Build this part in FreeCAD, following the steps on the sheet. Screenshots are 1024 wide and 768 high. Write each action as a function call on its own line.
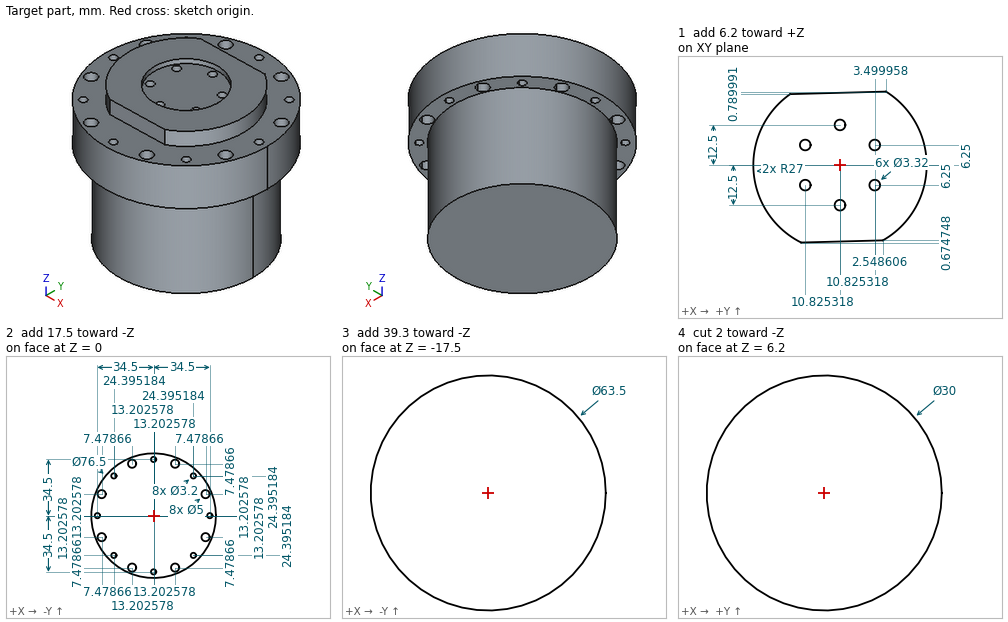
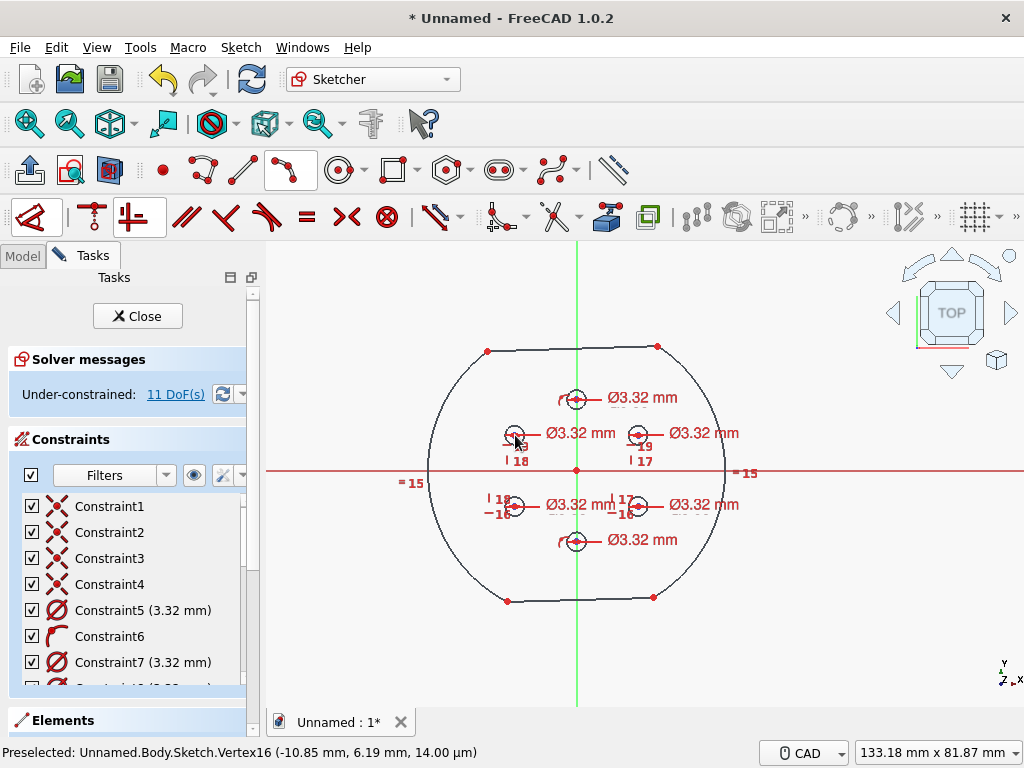
key(d)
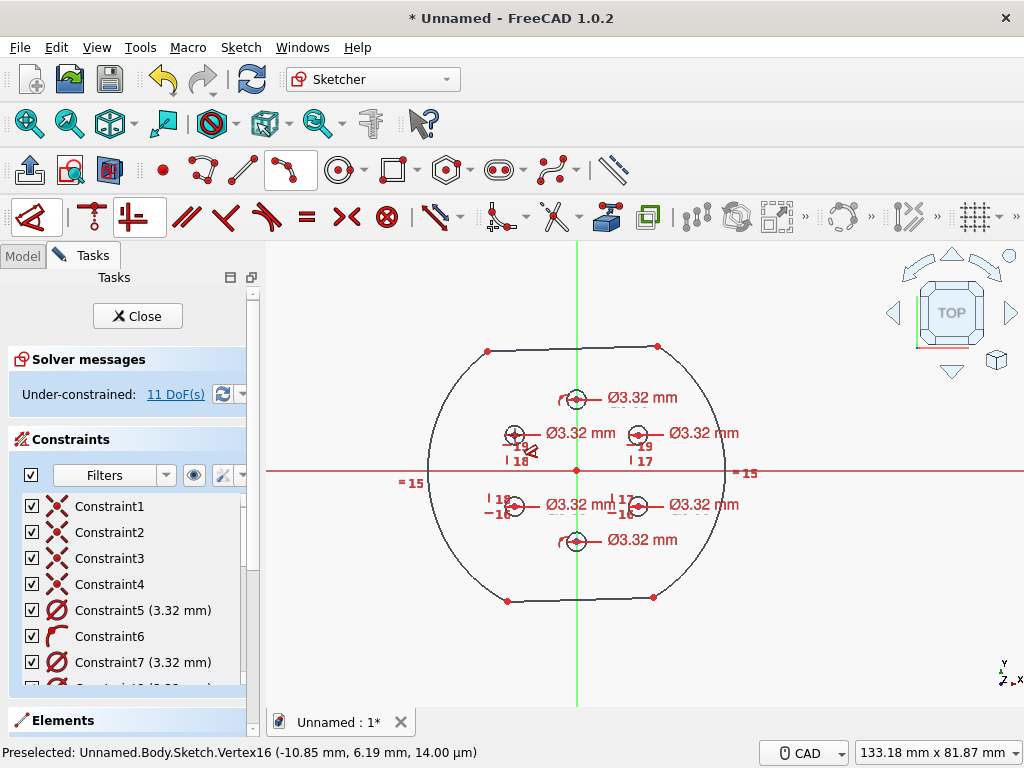
click(436, 423)
click(406, 413)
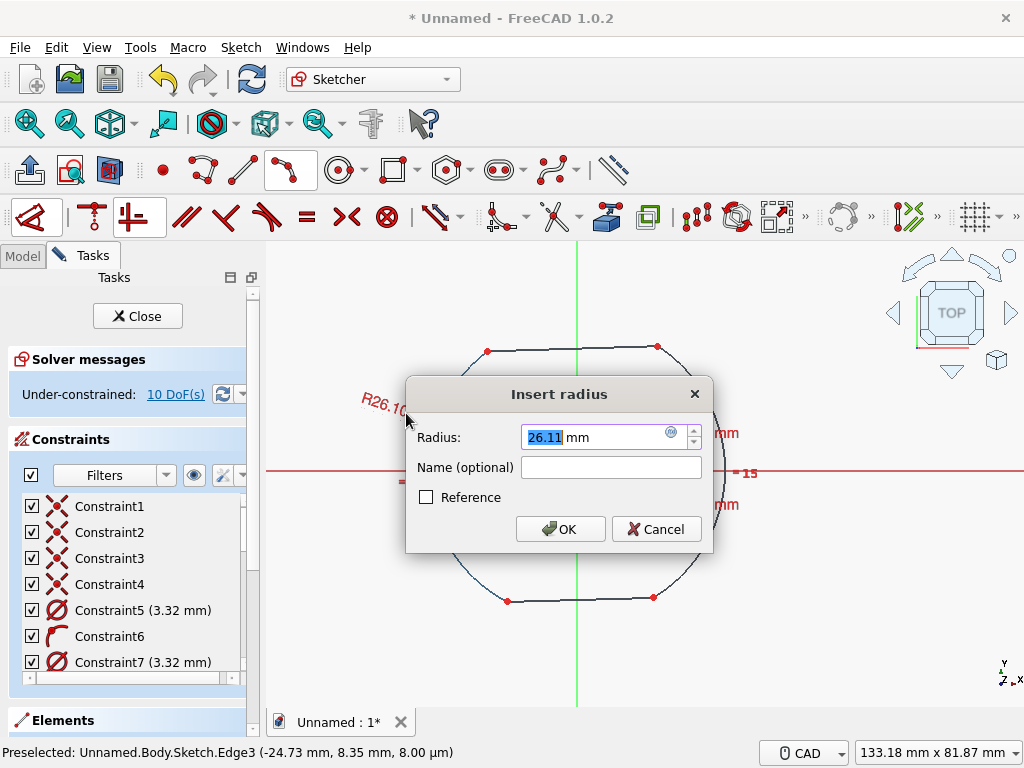
text(27)
key(Return)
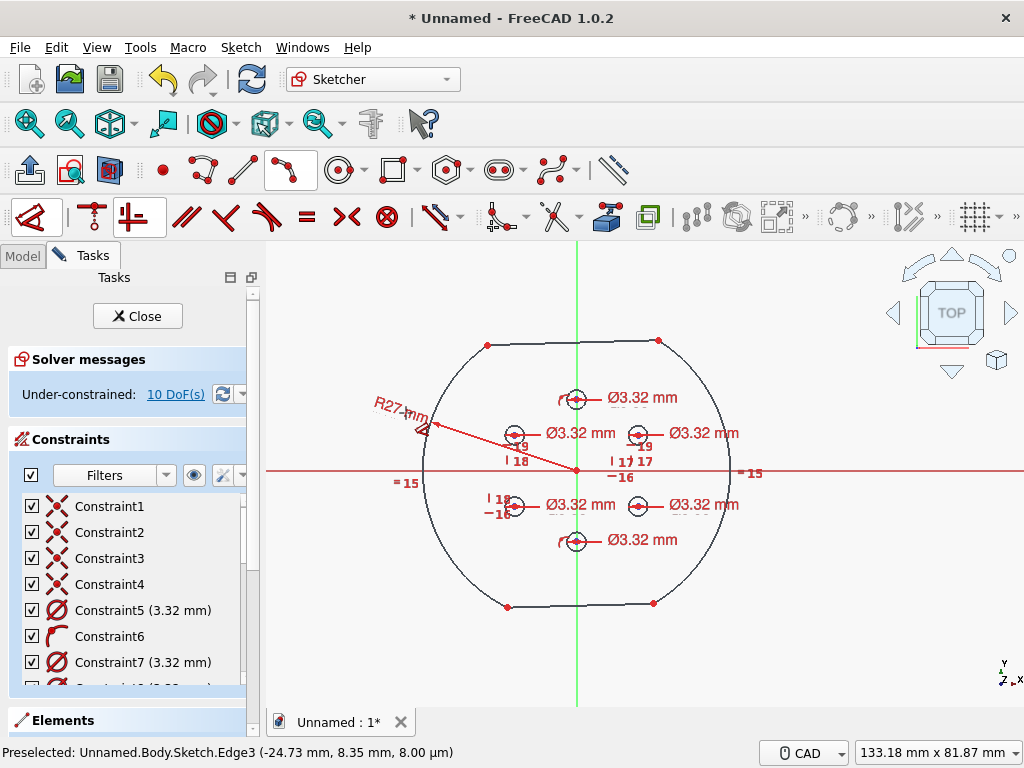
click(577, 542)
click(543, 506)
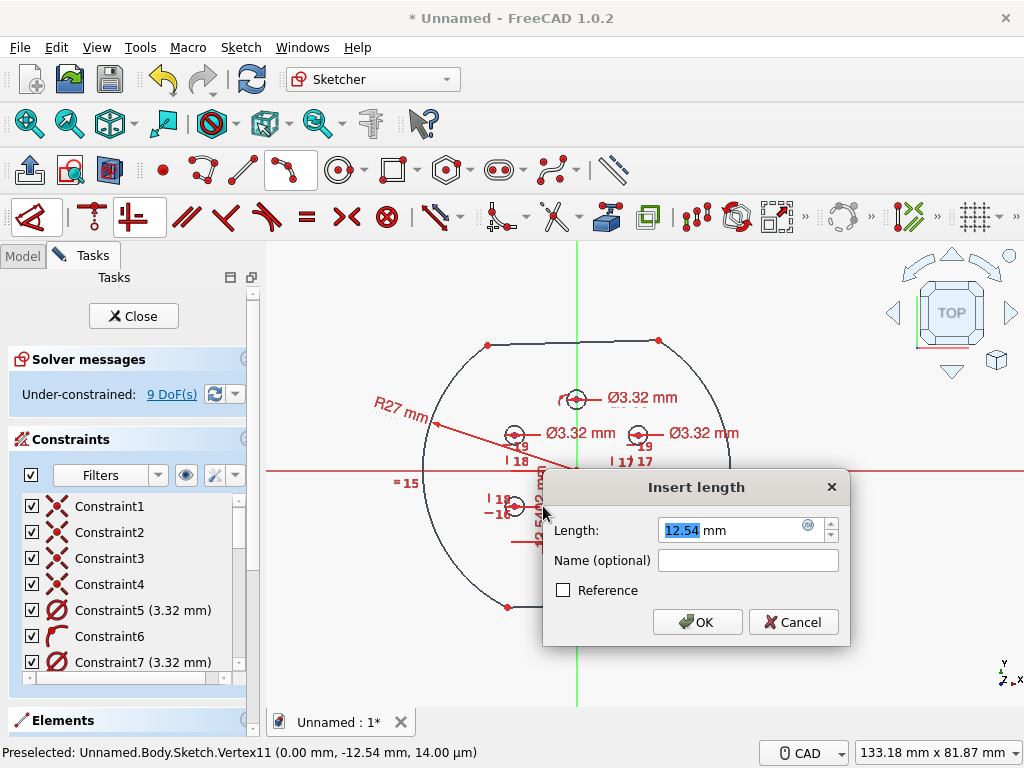
text(12.5)
key(Return)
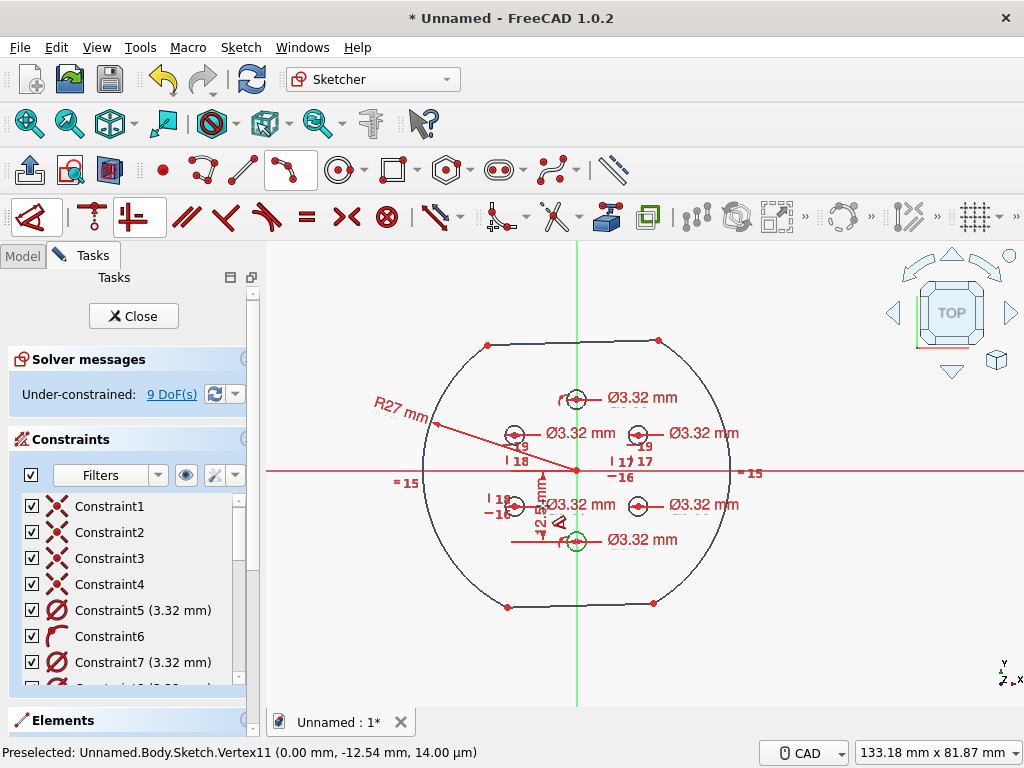
click(638, 507)
click(672, 489)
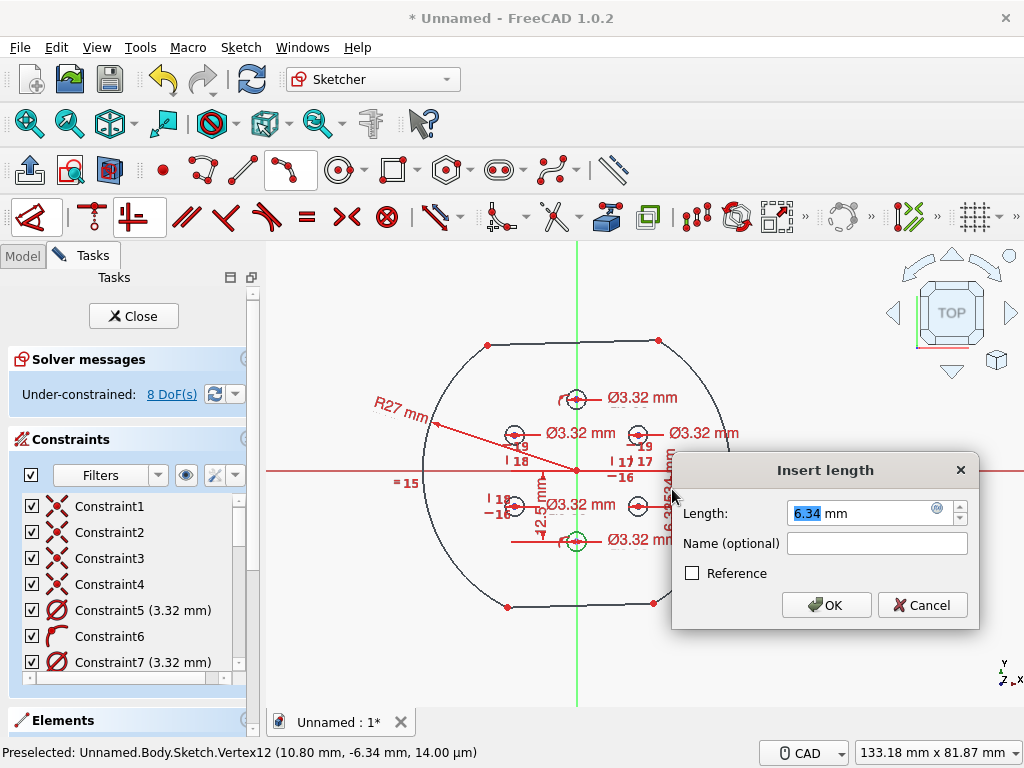
text(6.25)
key(Return)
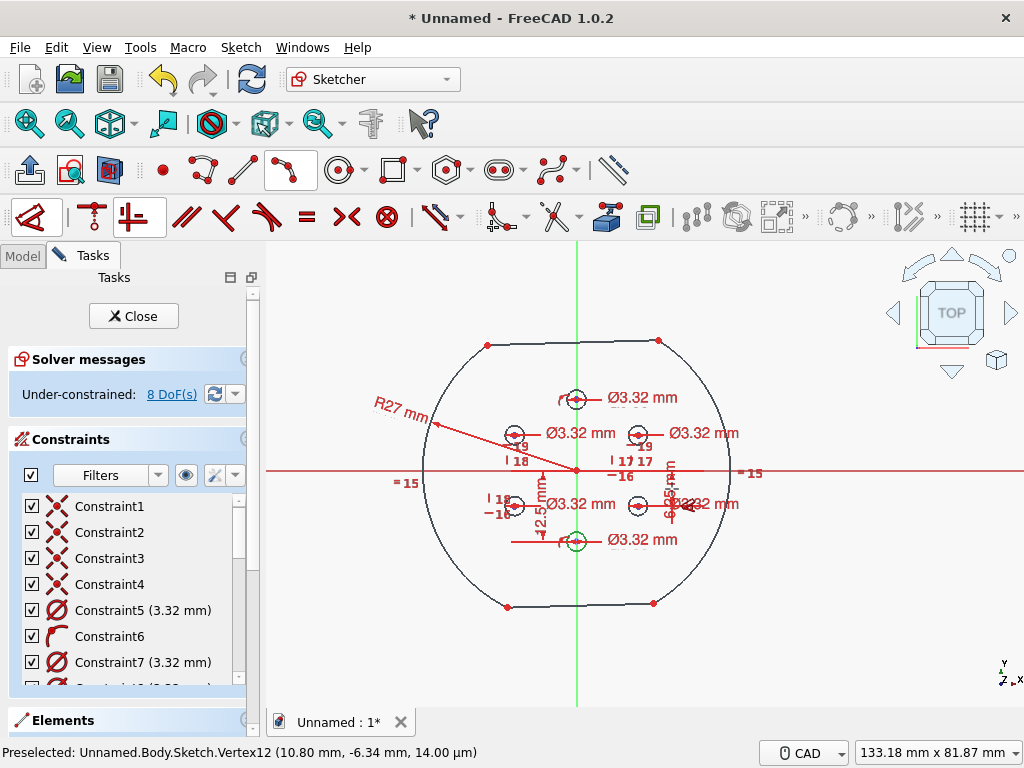
click(638, 435)
click(672, 453)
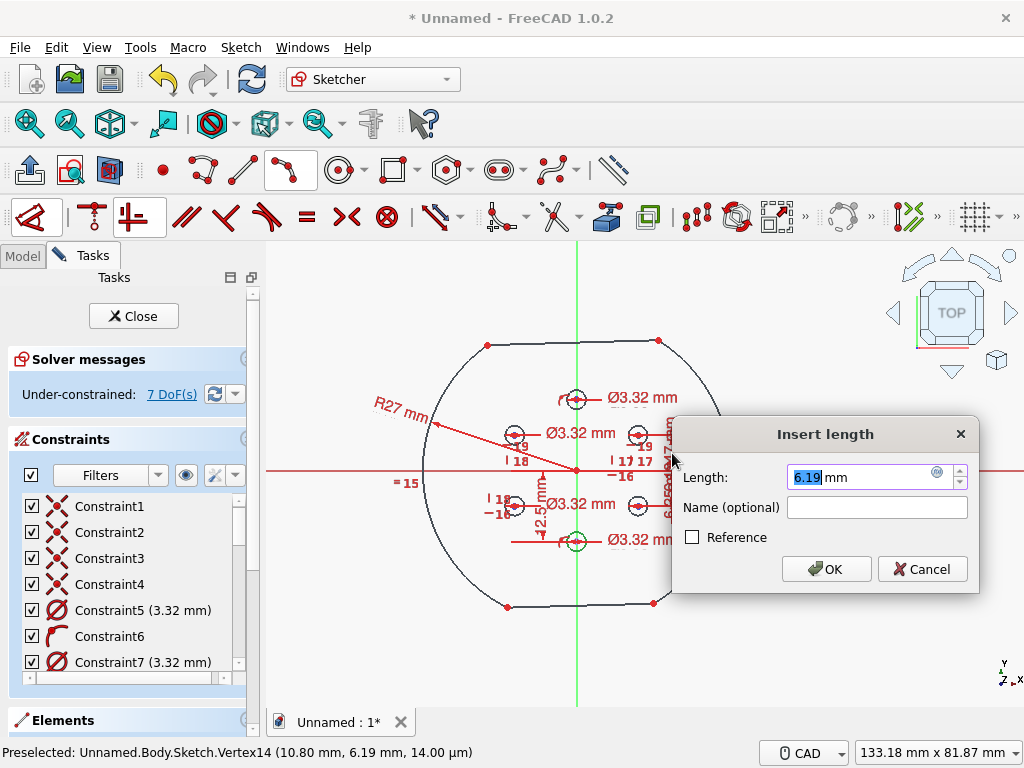
text(6.25)
key(Return)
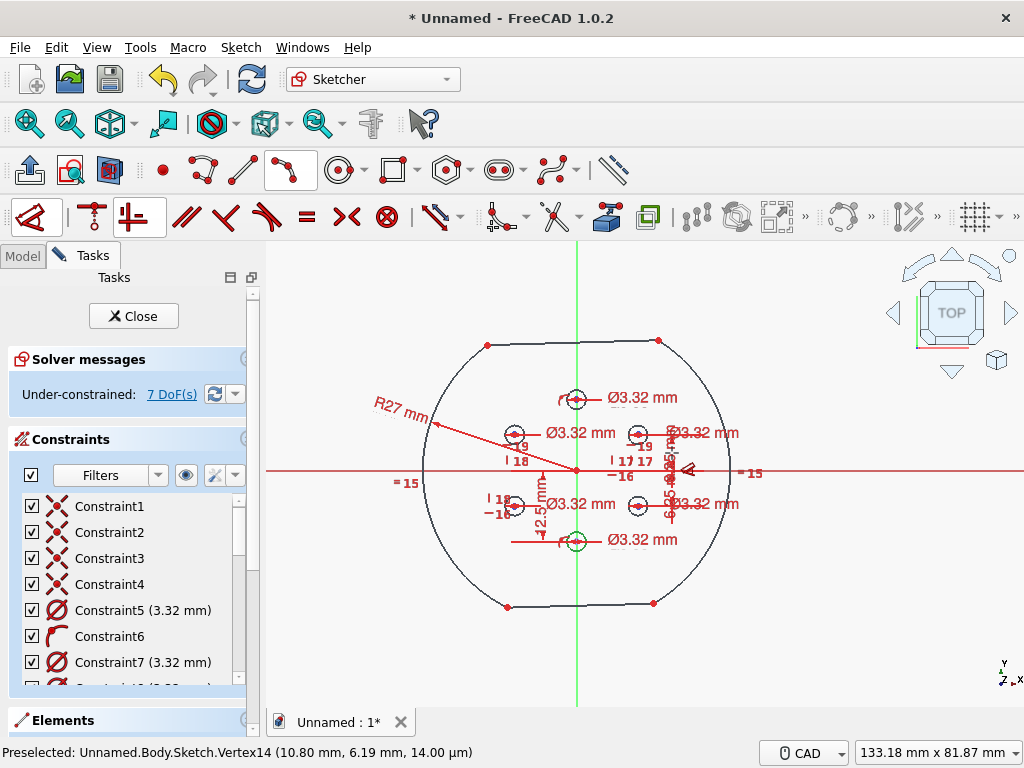
click(577, 400)
click(543, 435)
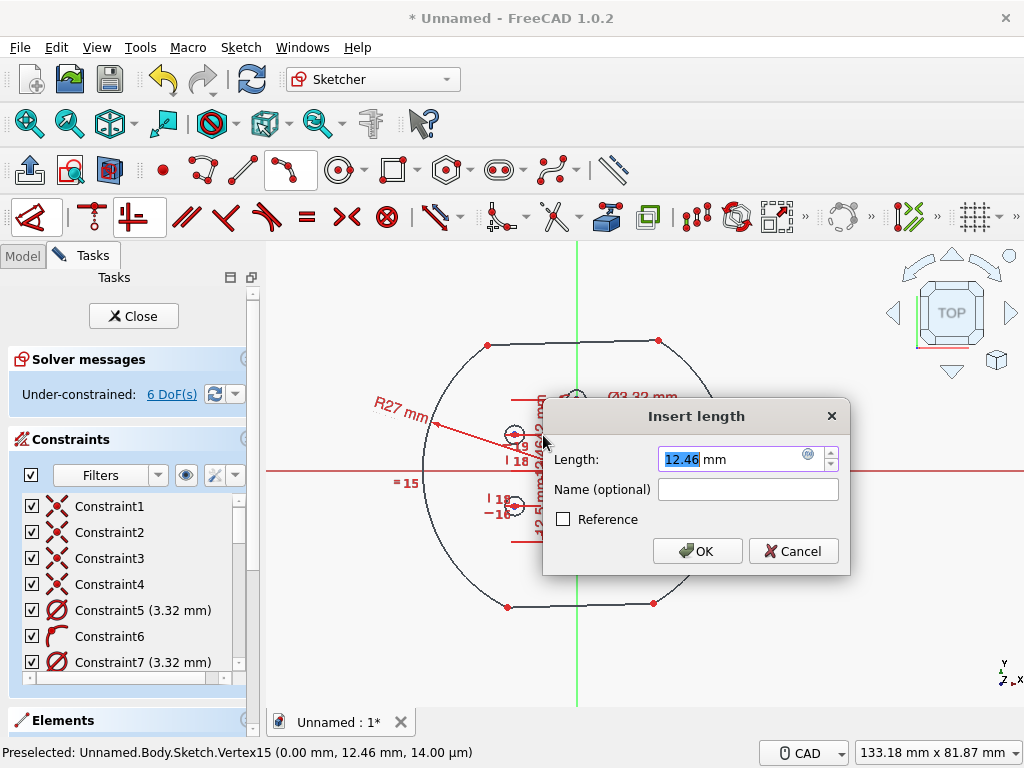
text(12.5)
key(Return)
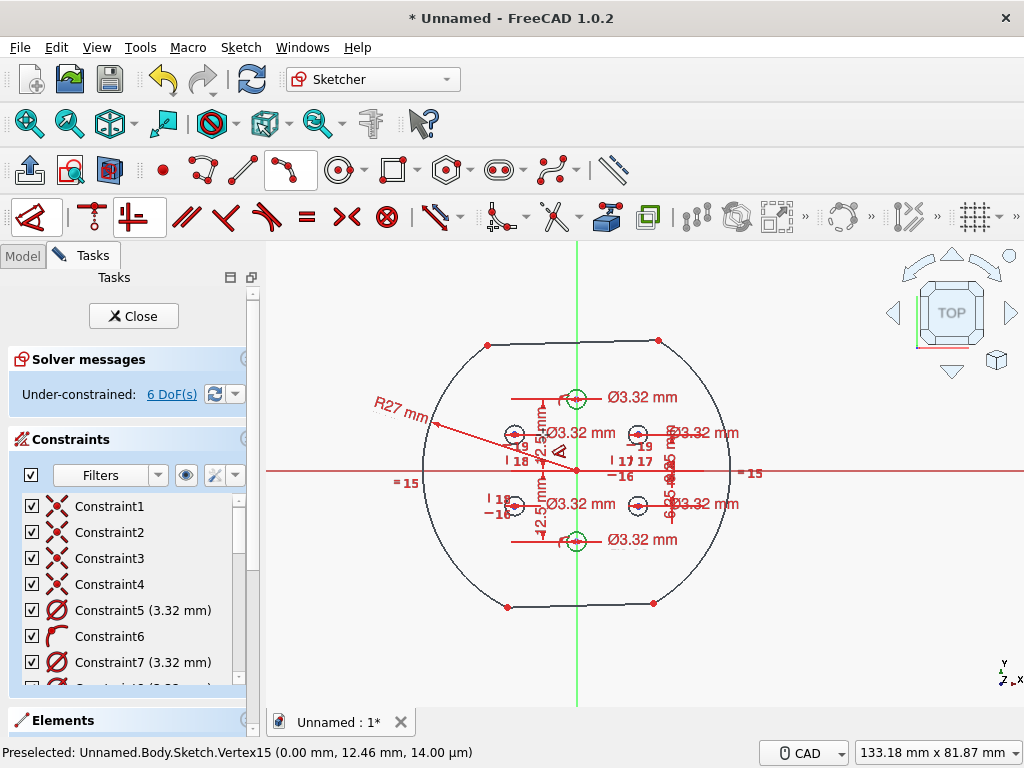
scroll(607, 342, up, 11)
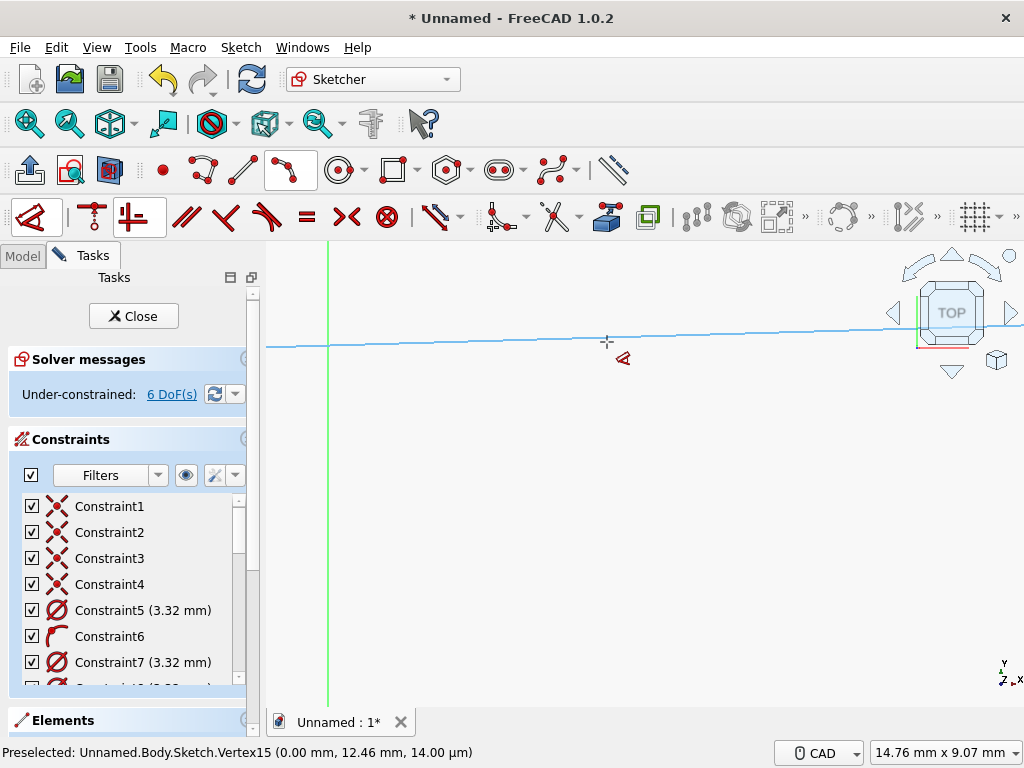
click(603, 338)